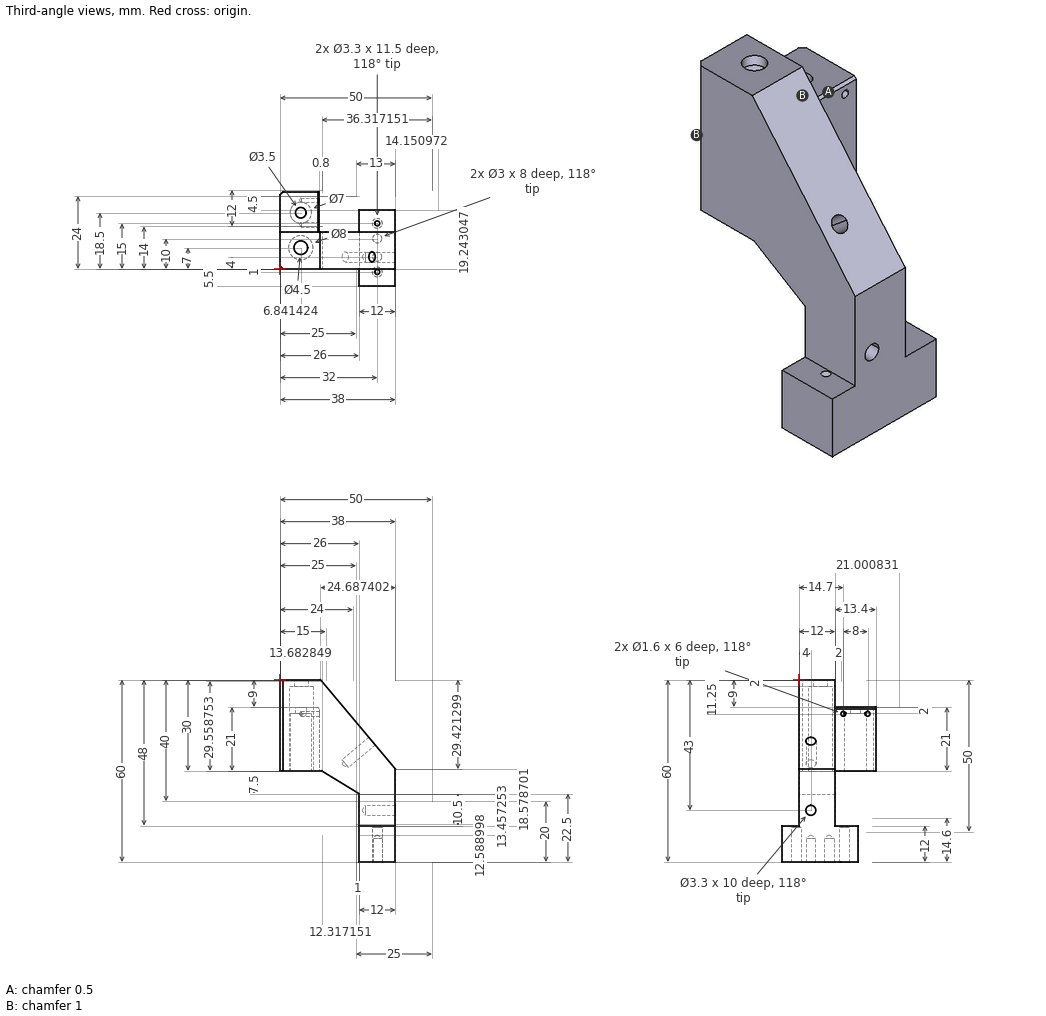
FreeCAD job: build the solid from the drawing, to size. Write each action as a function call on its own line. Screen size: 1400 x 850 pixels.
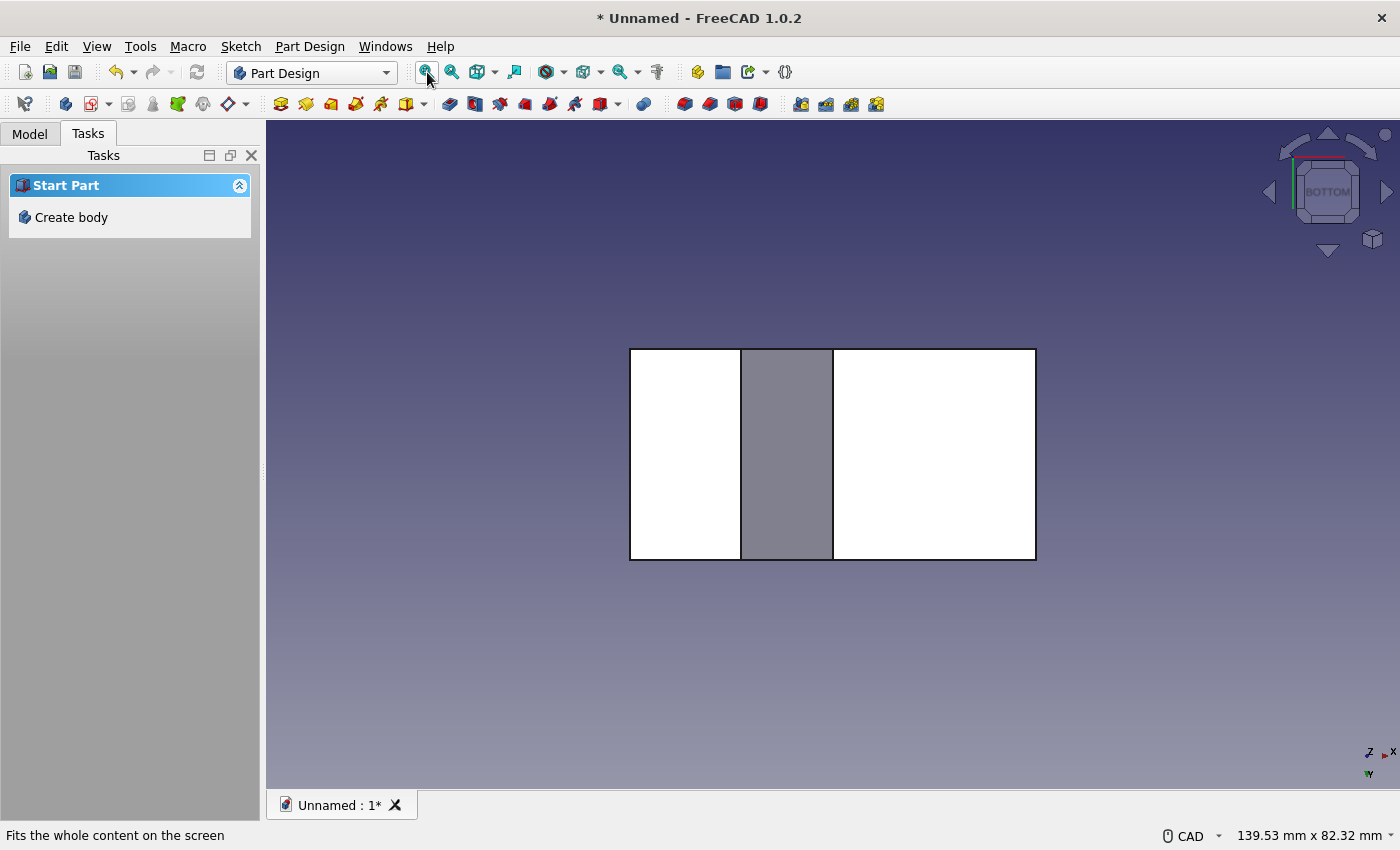
click(427, 72)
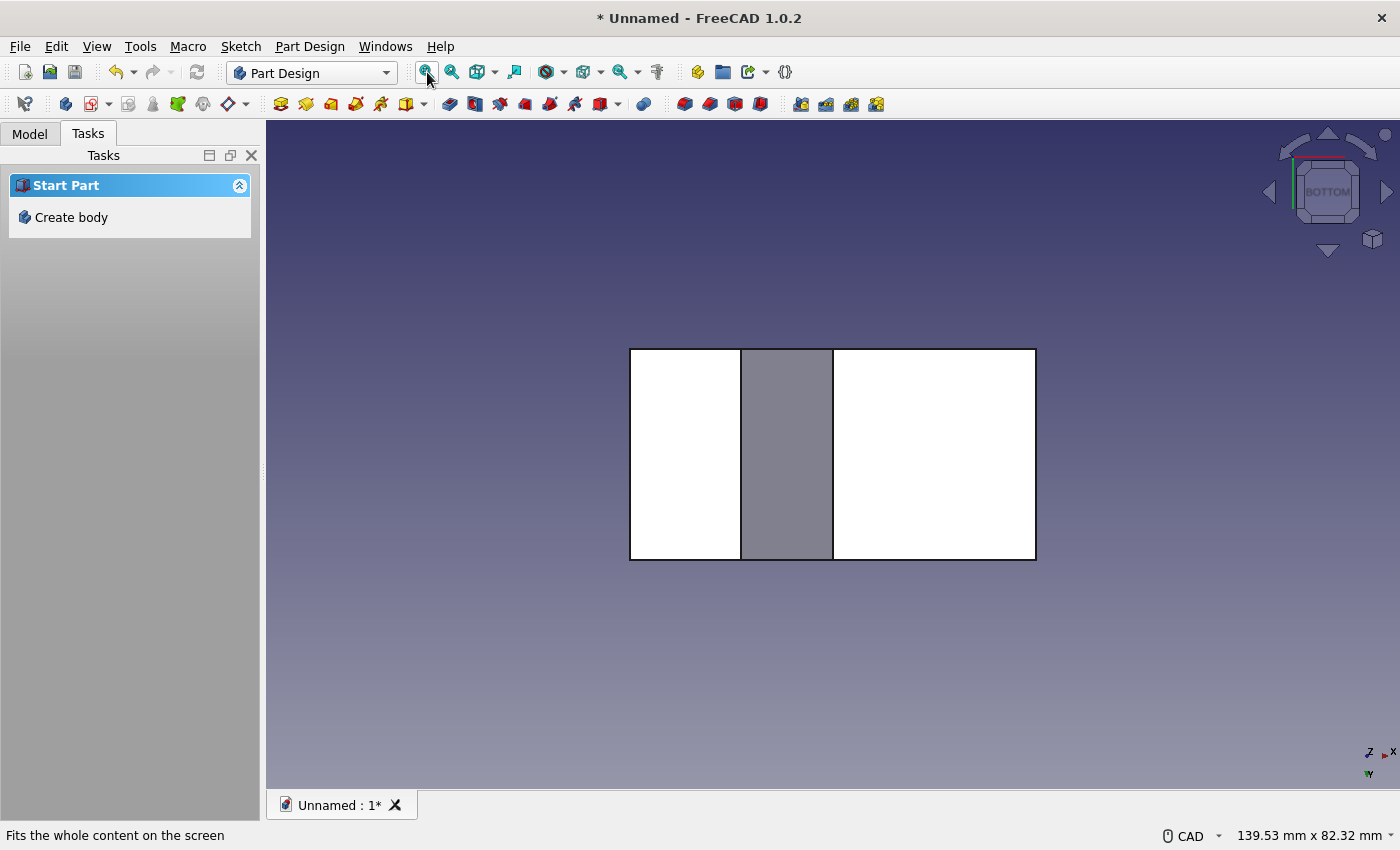
click(935, 453)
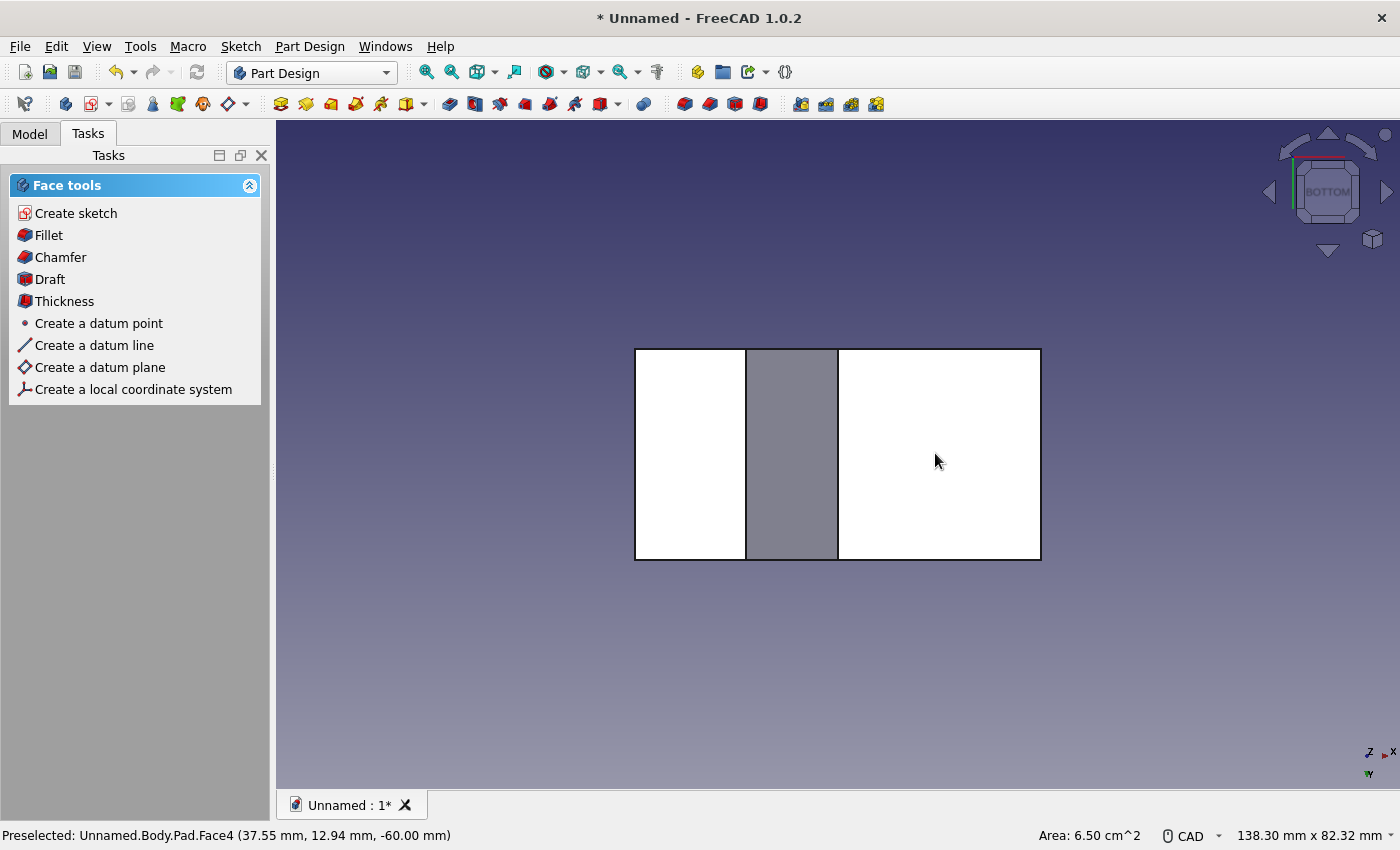
click(90, 104)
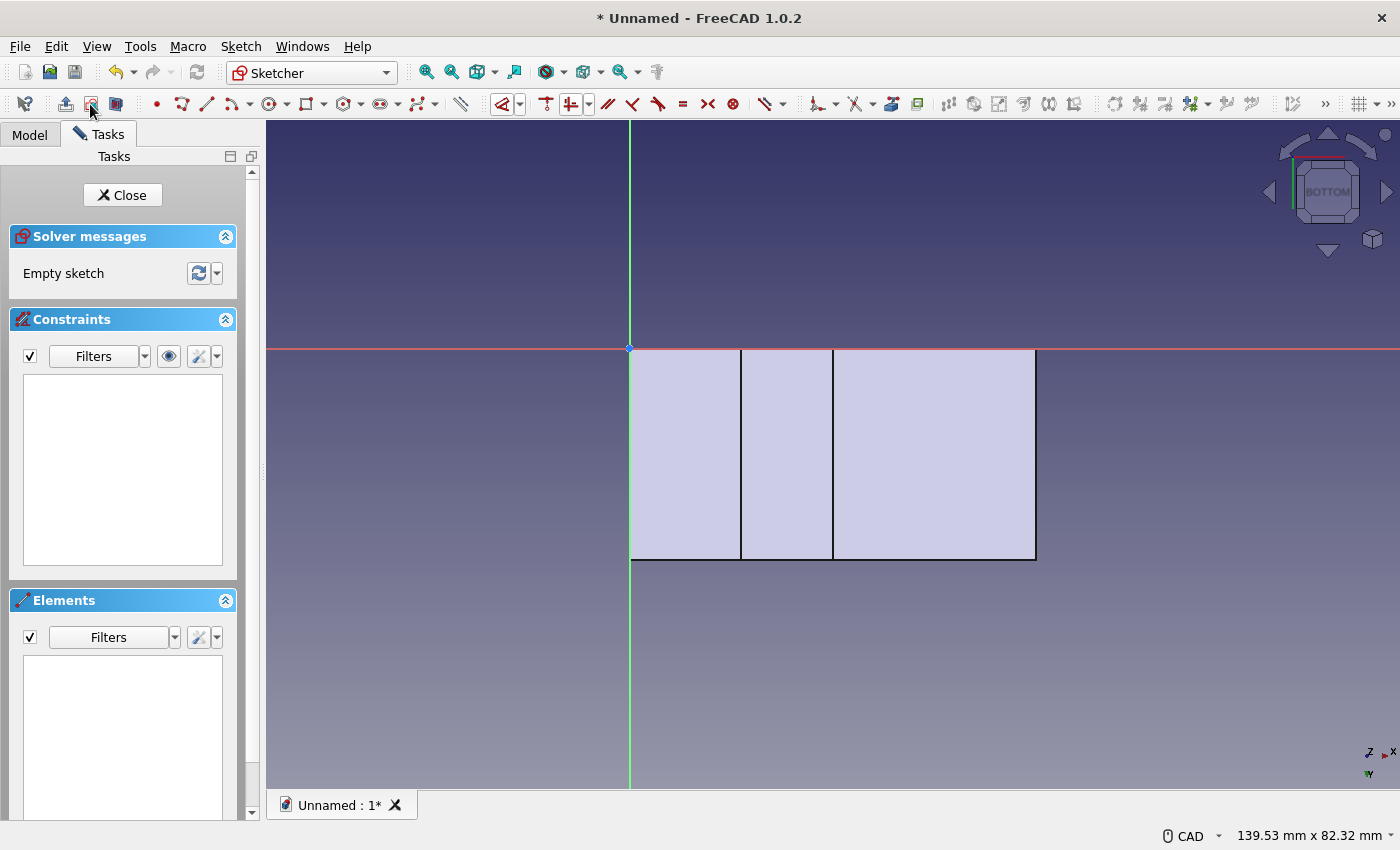
scroll(972, 454, up, 2)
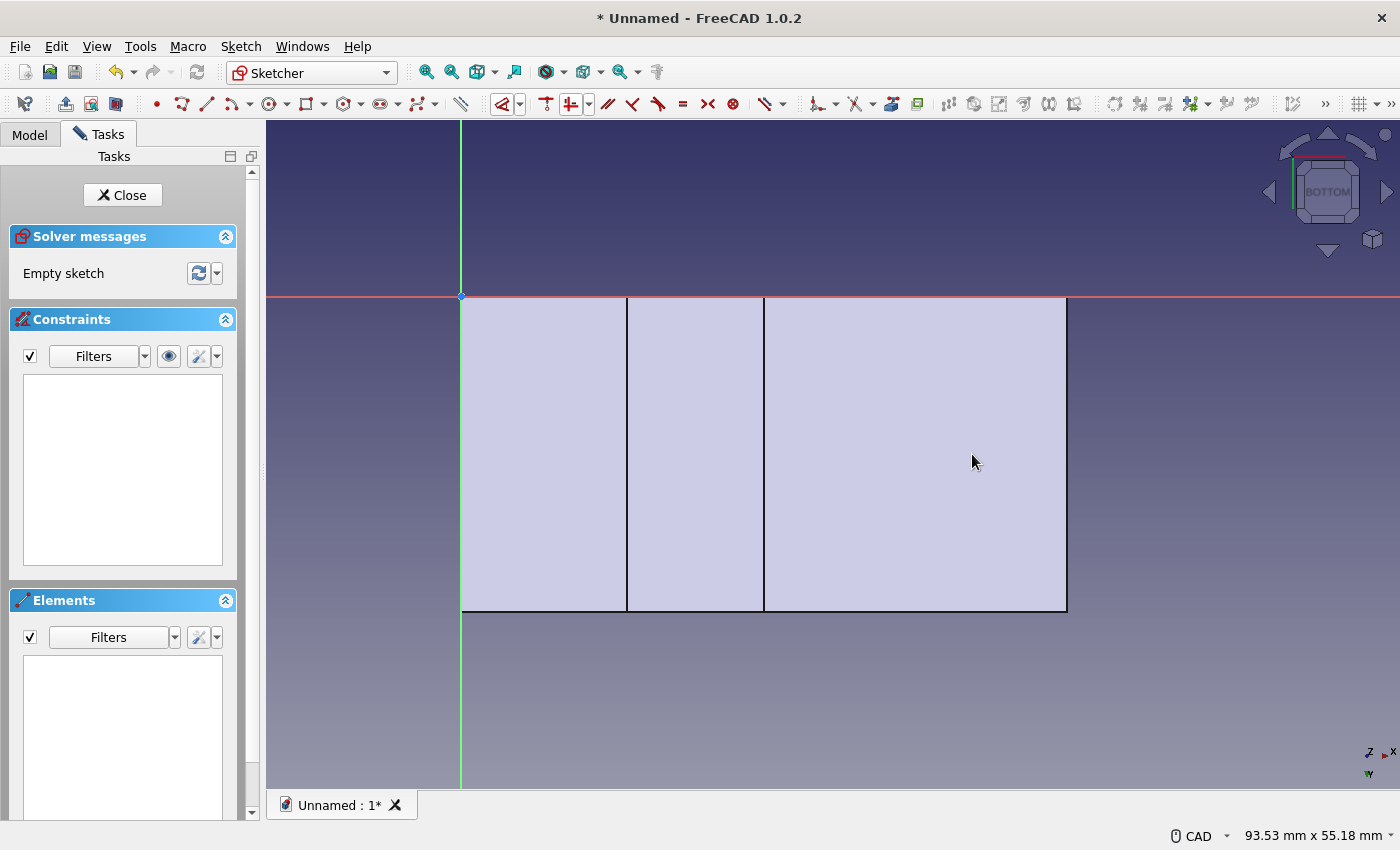
click(306, 104)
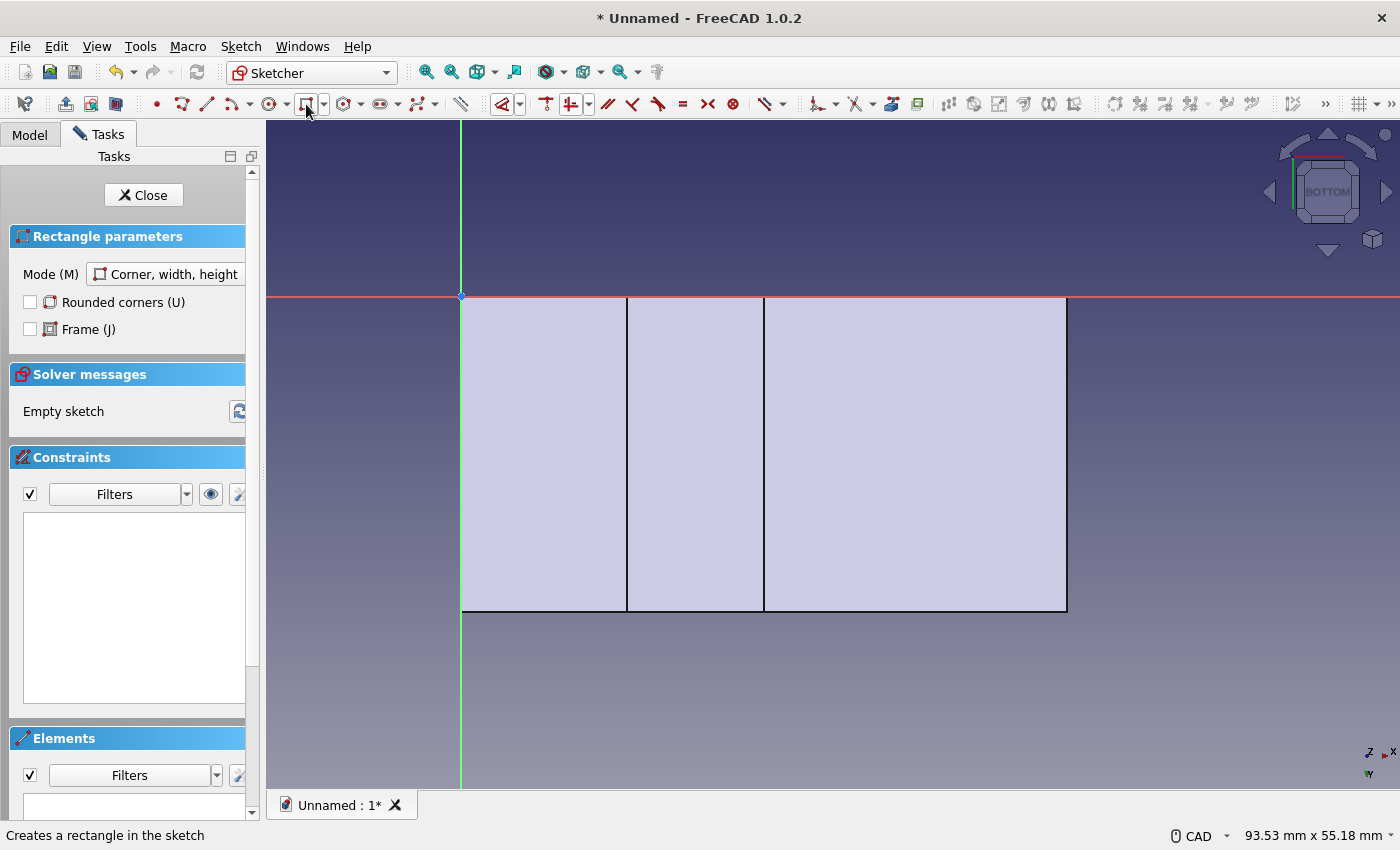
click(627, 467)
click(1067, 612)
key(Escape)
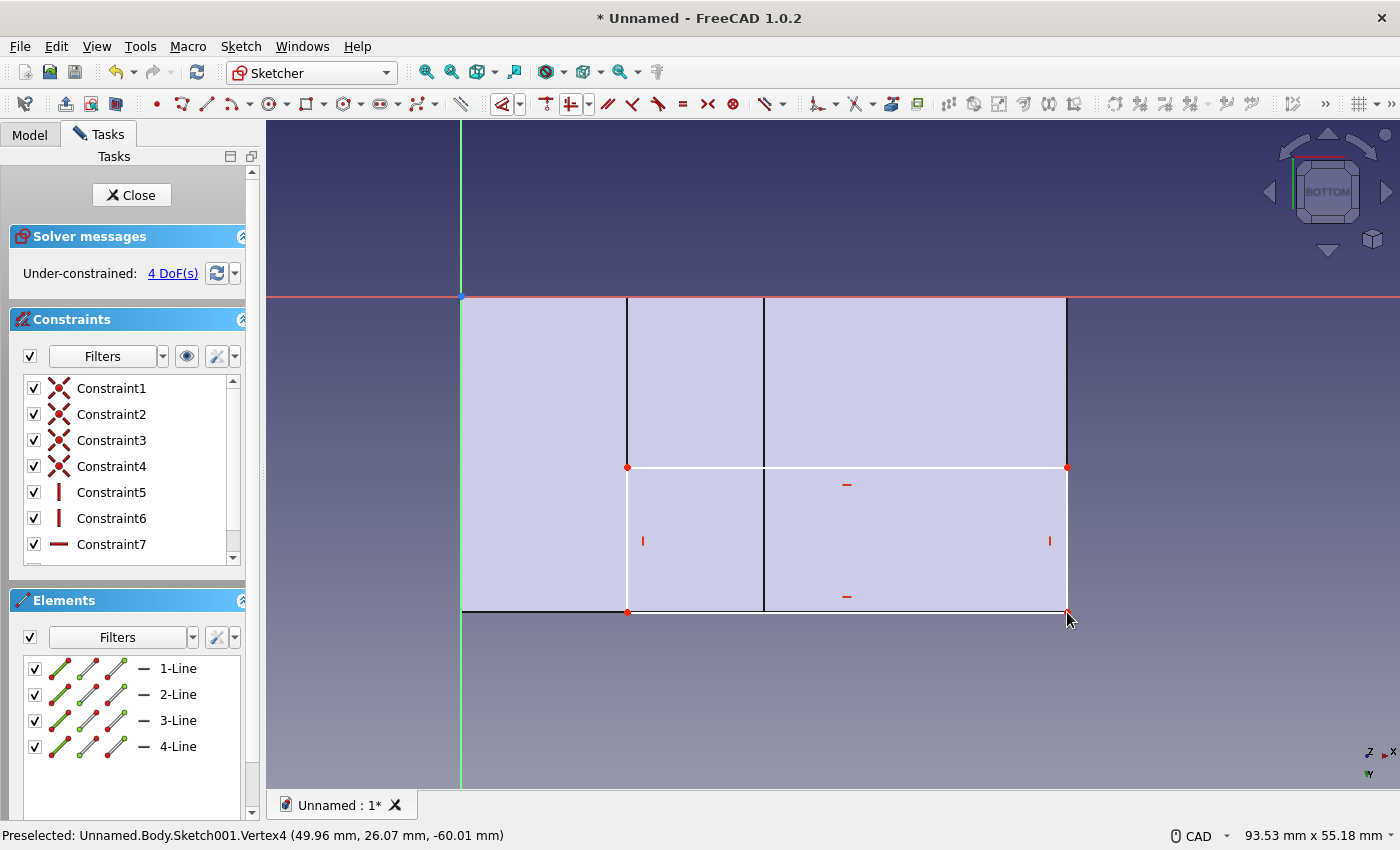
click(627, 511)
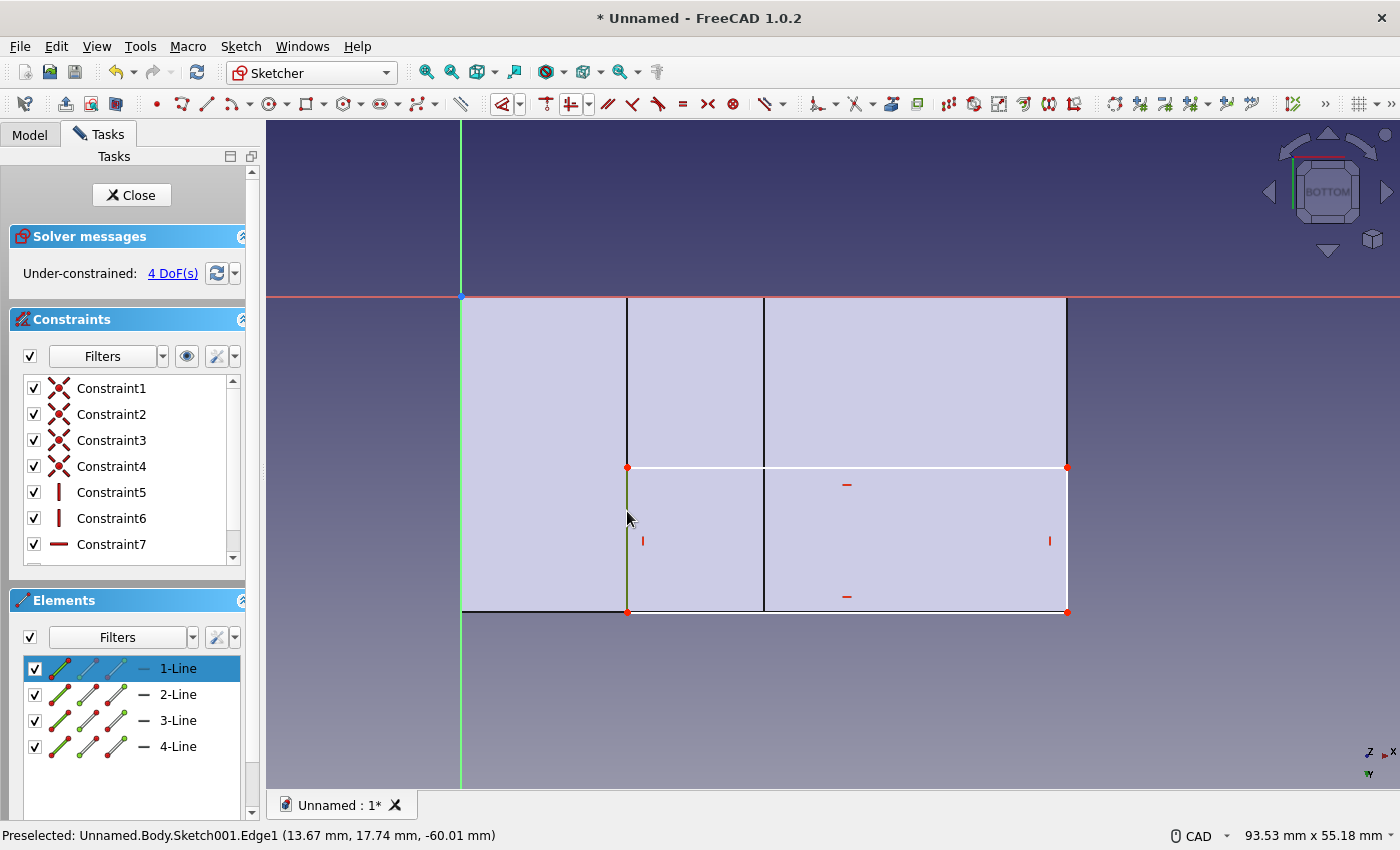
click(520, 104)